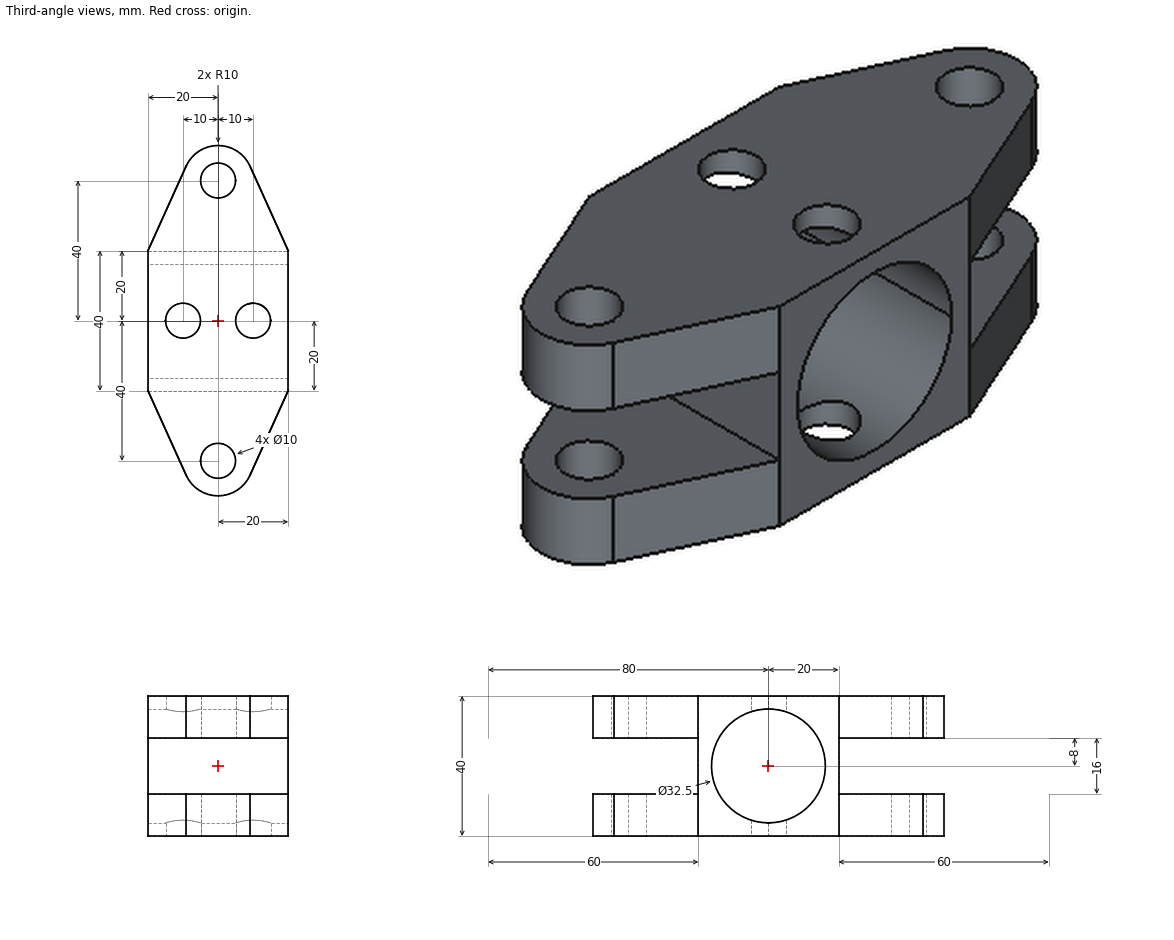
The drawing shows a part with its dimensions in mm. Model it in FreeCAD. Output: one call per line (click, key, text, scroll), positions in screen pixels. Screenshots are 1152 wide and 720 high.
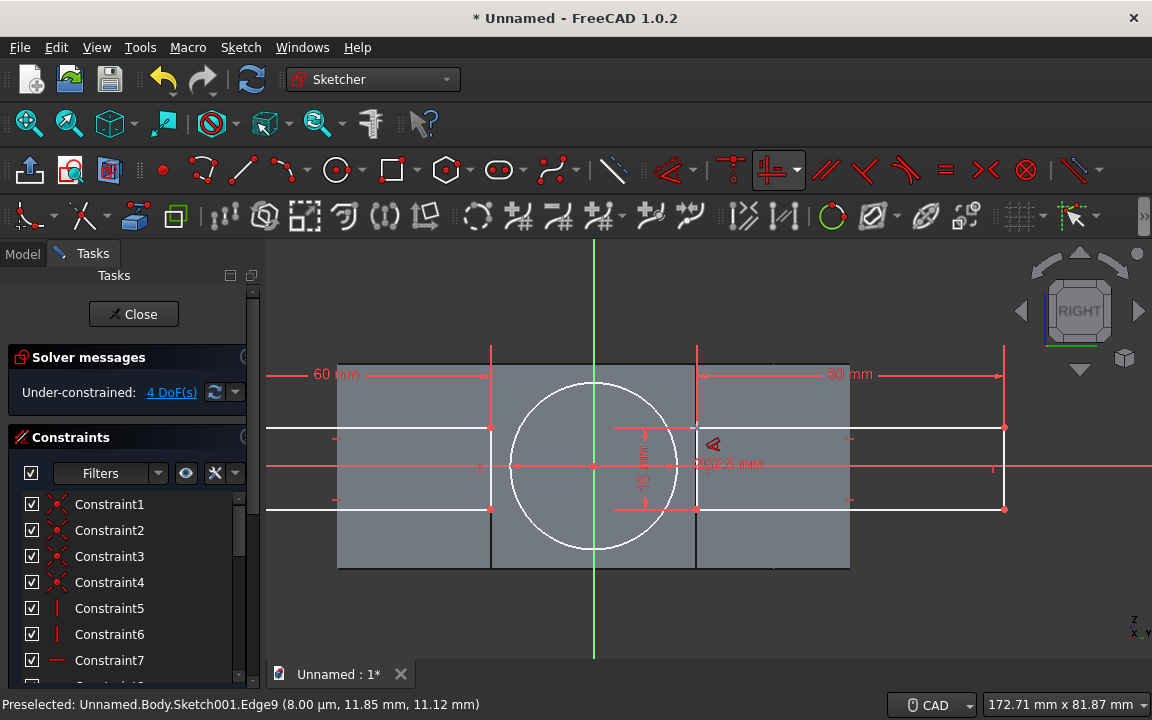
click(697, 428)
click(731, 447)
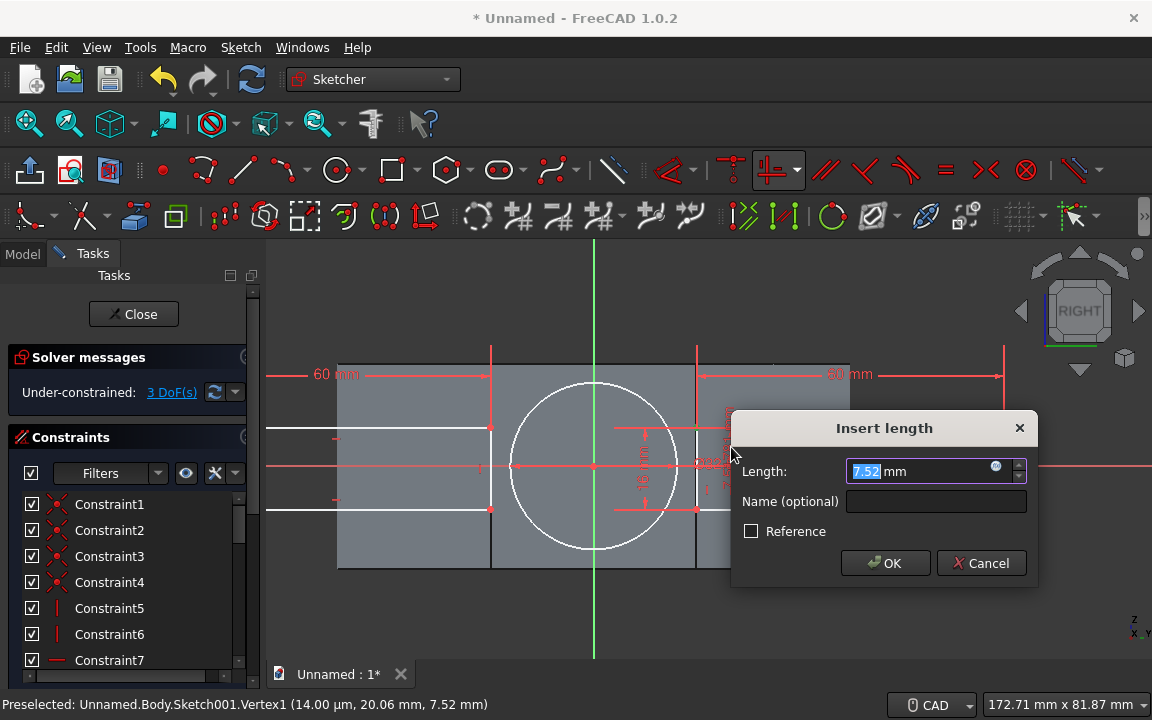
text(8)
key(Return)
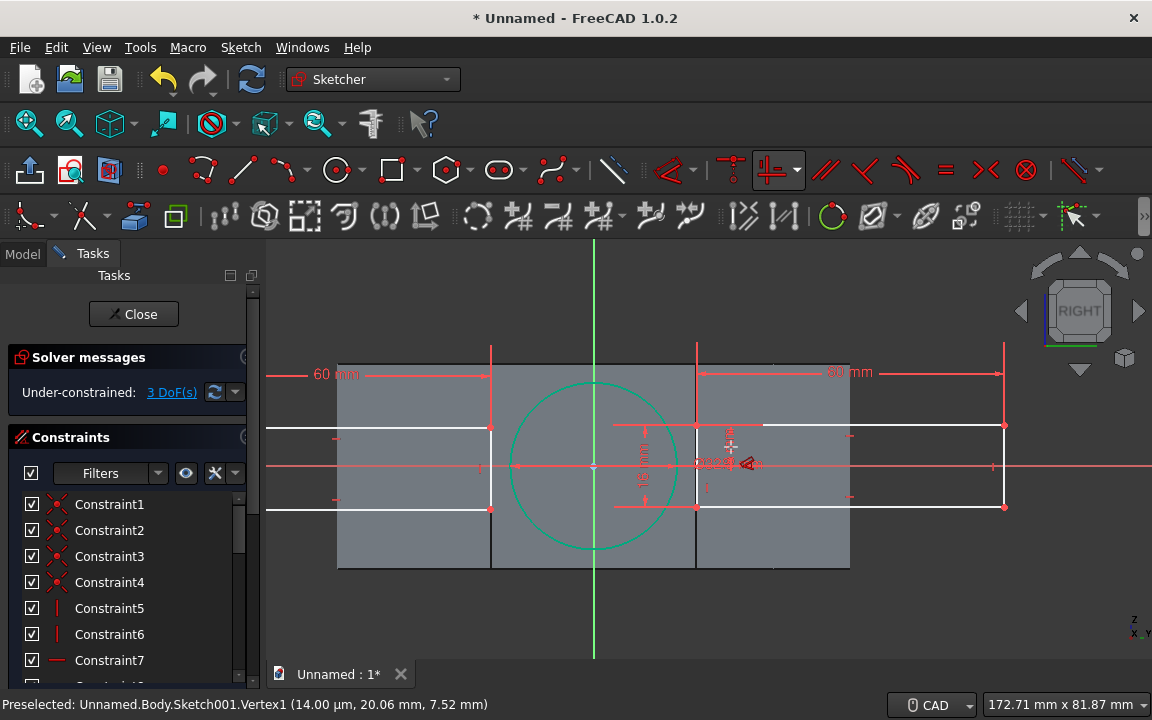
scroll(697, 428, down, 3)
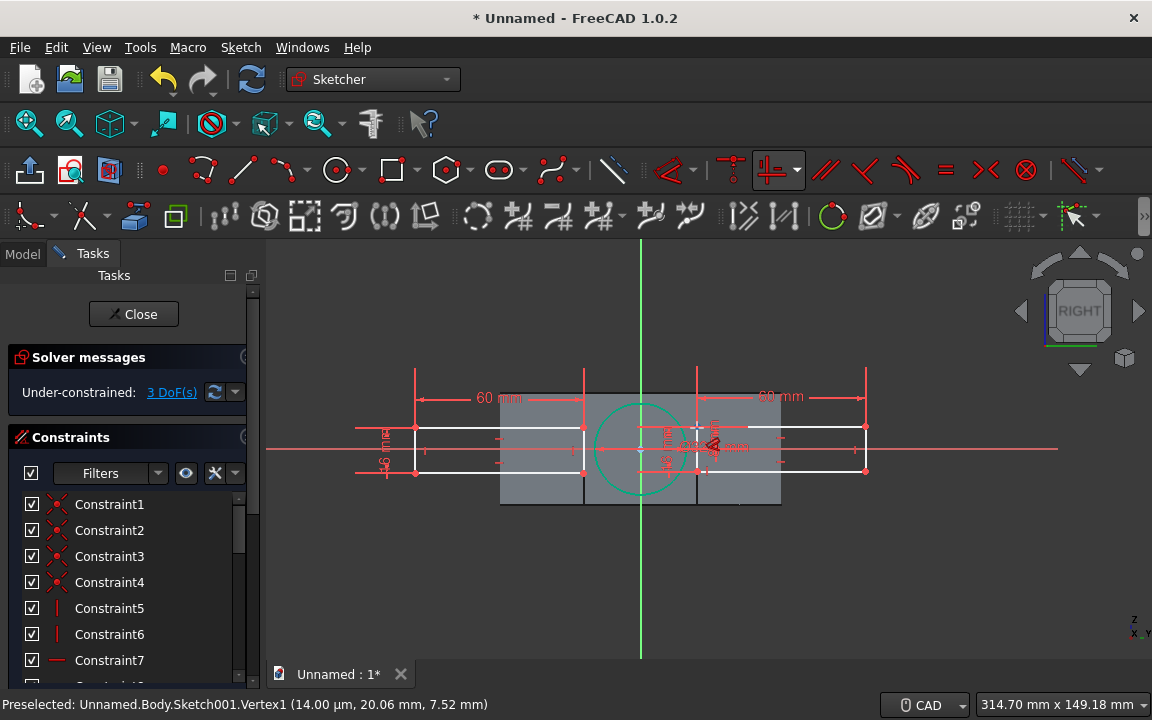
scroll(415, 428, up, 3)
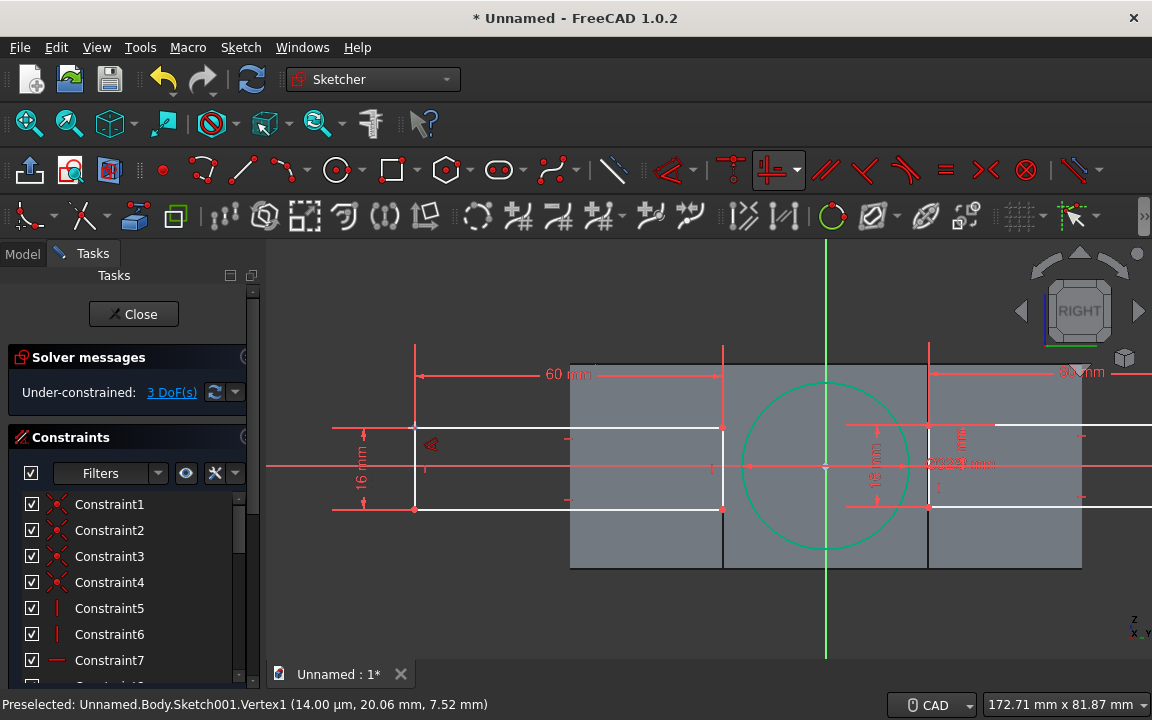
click(415, 428)
click(381, 447)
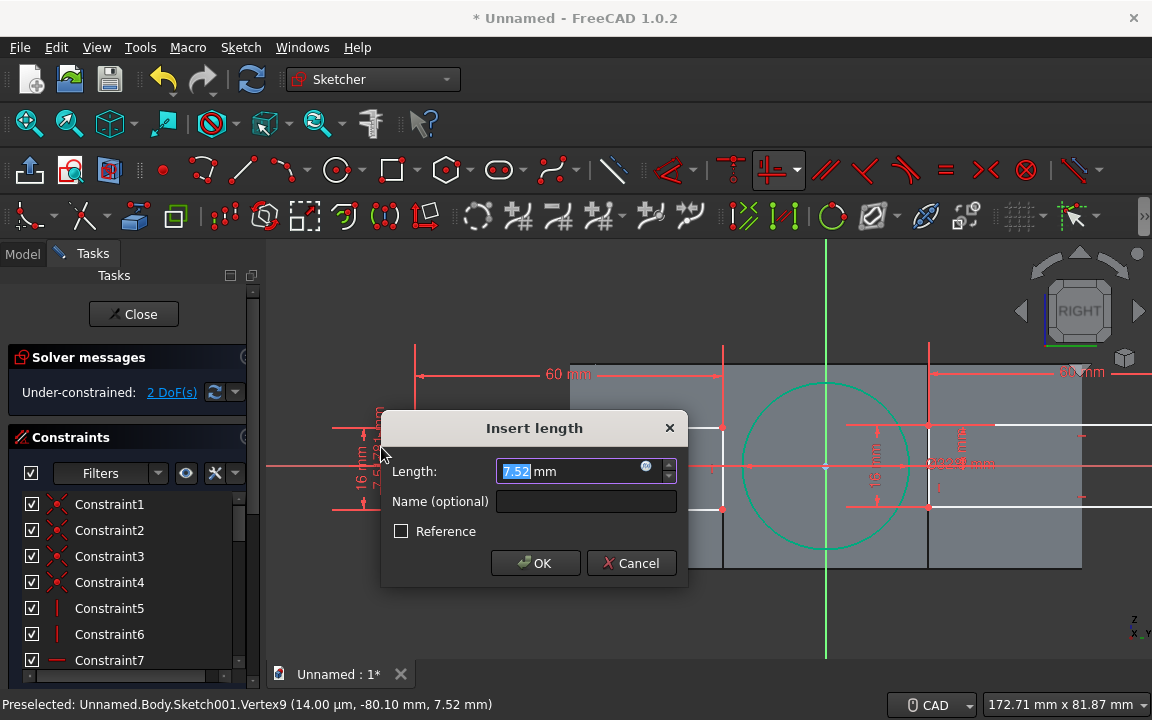
text(8)
key(Return)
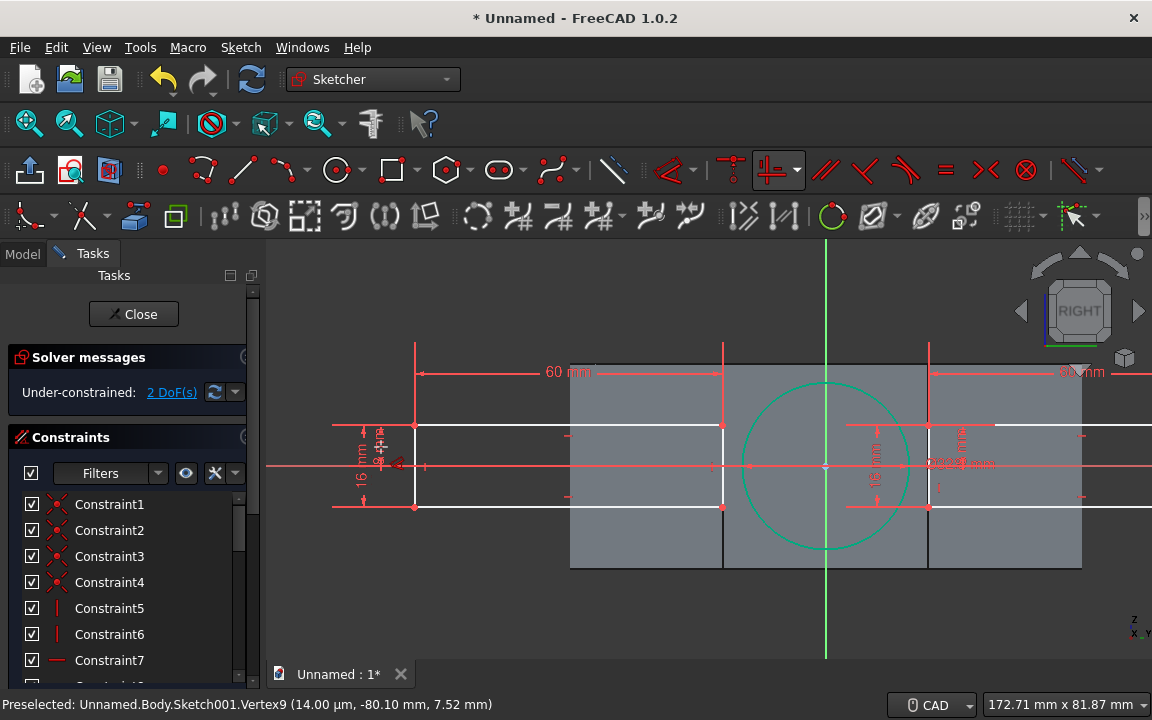
click(929, 425)
click(901, 391)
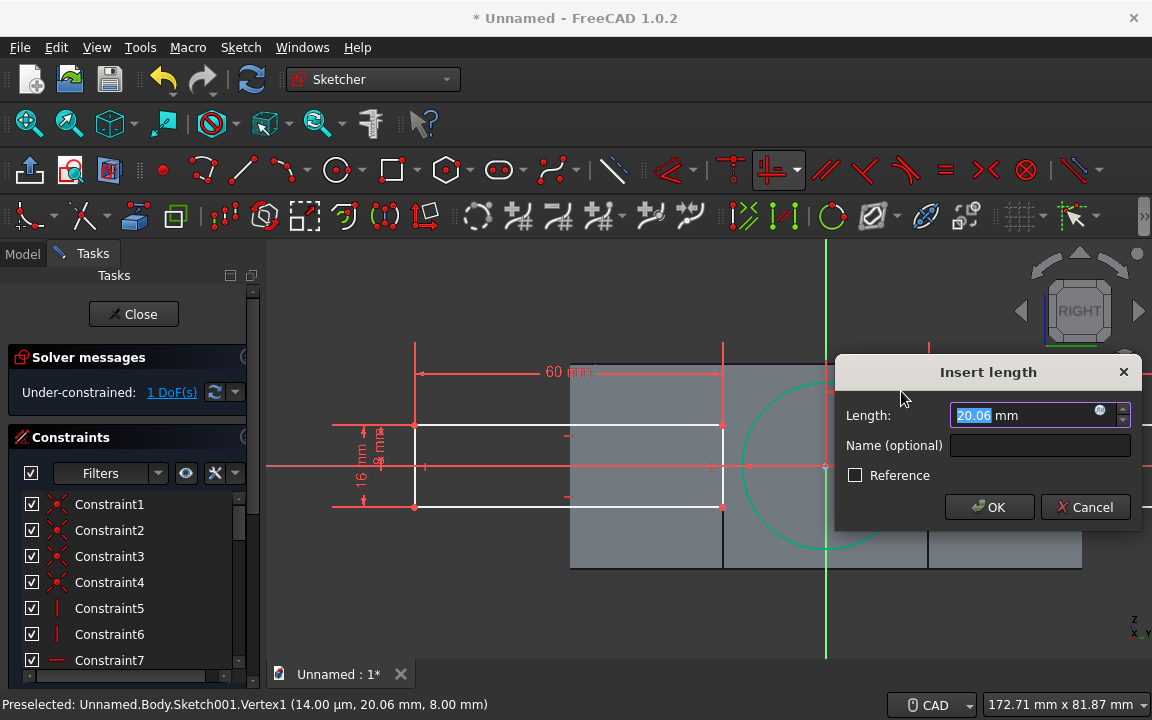
text(20)
key(Return)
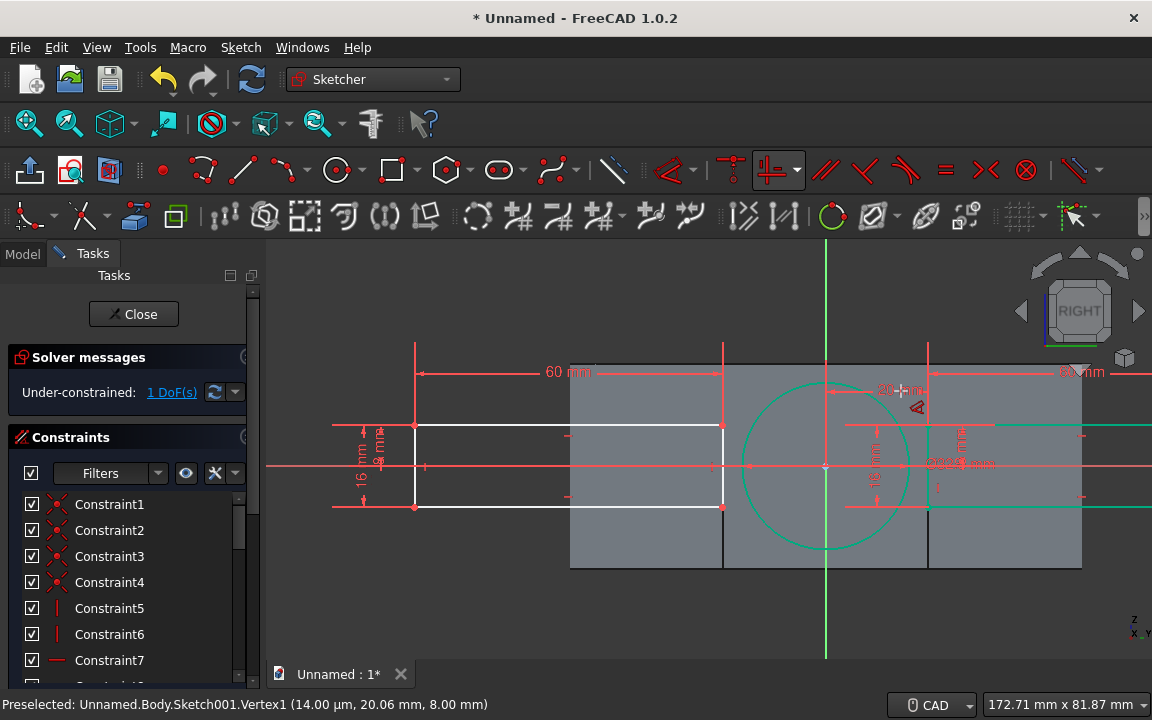
click(415, 425)
click(620, 391)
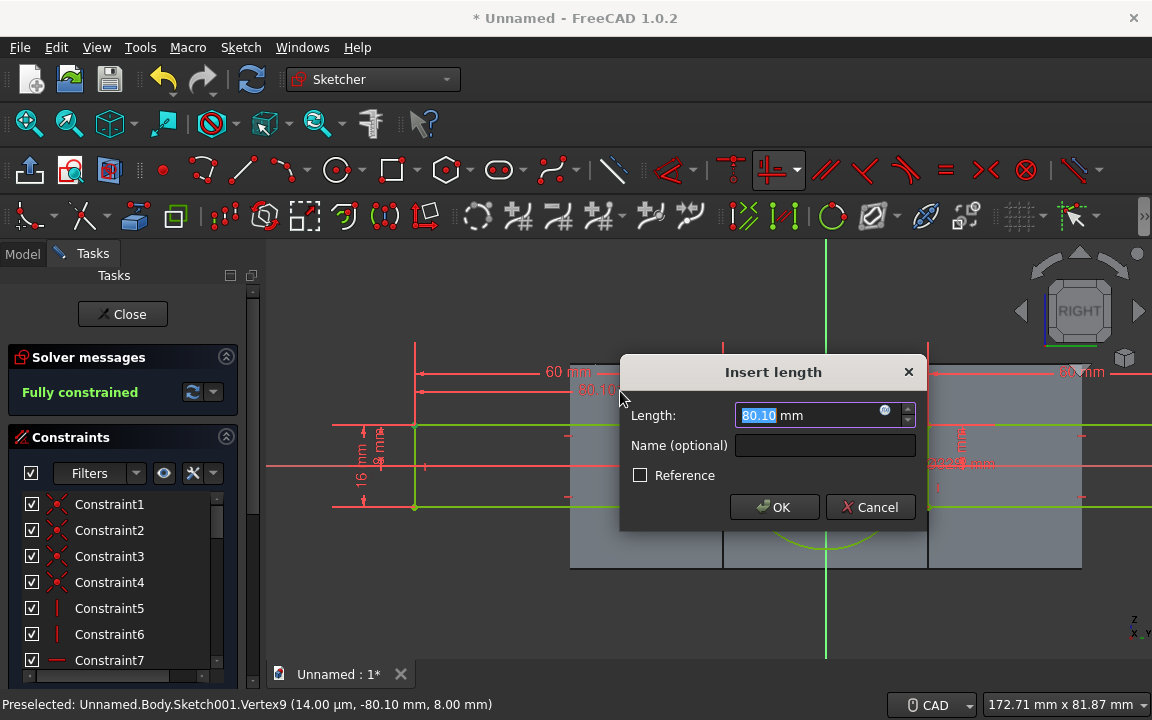
text(80)
key(Return)
key(Escape)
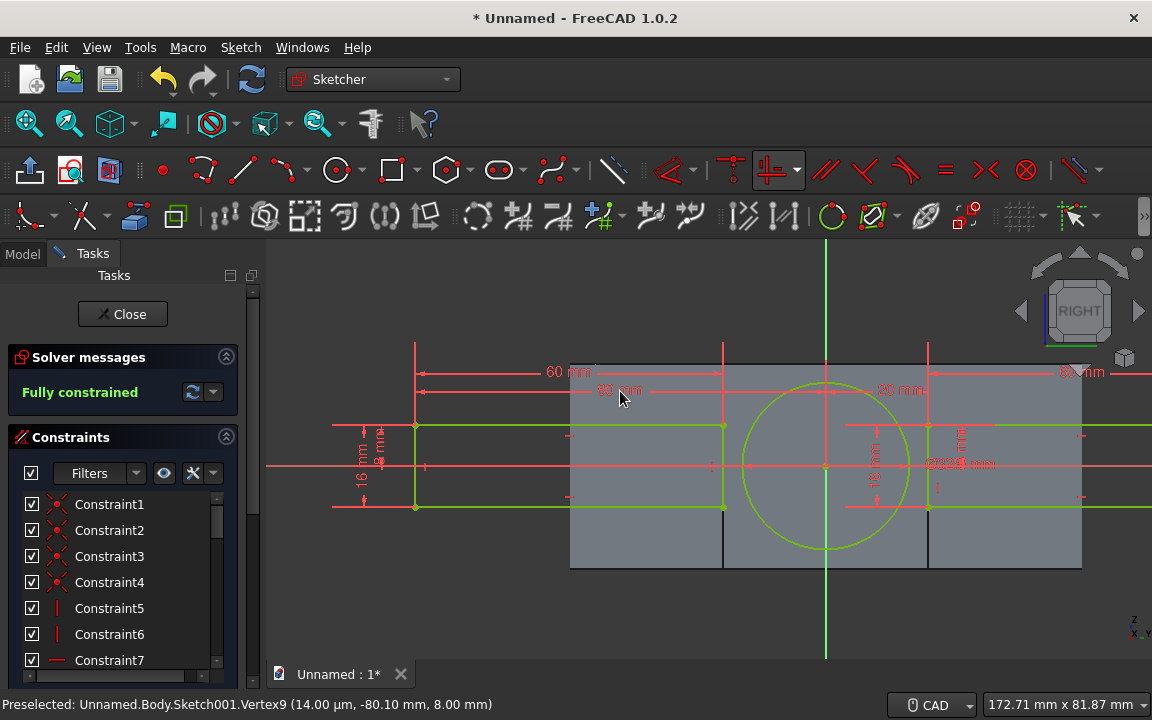
click(123, 314)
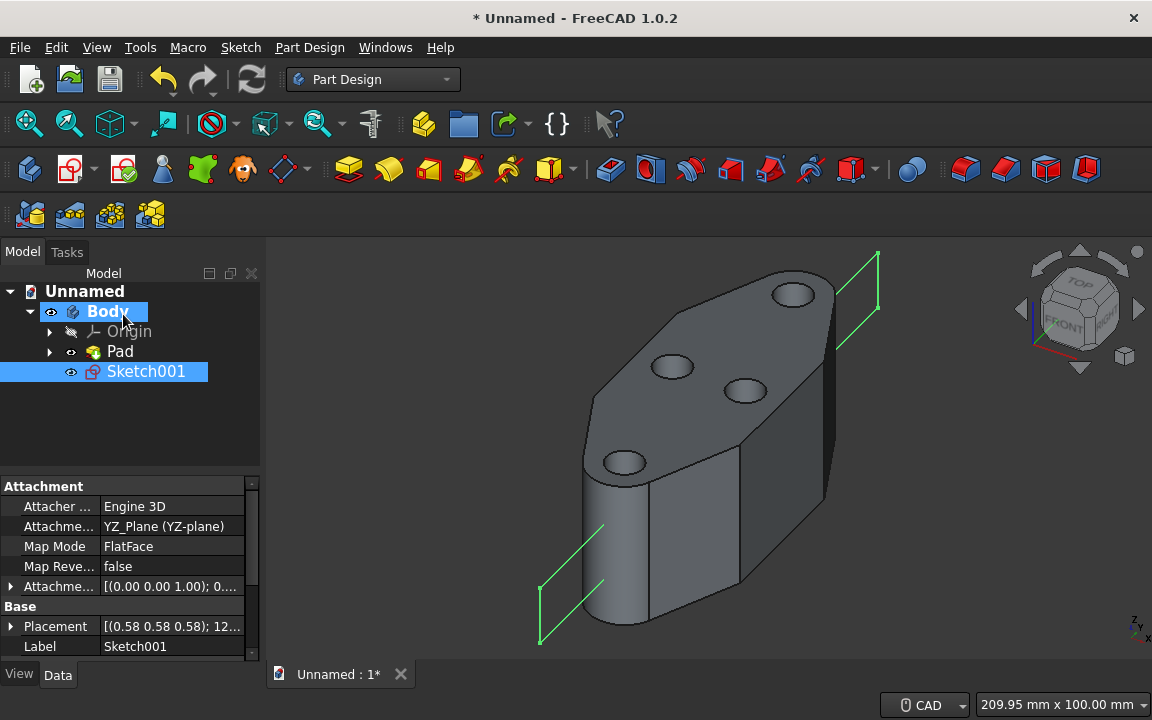
click(612, 170)